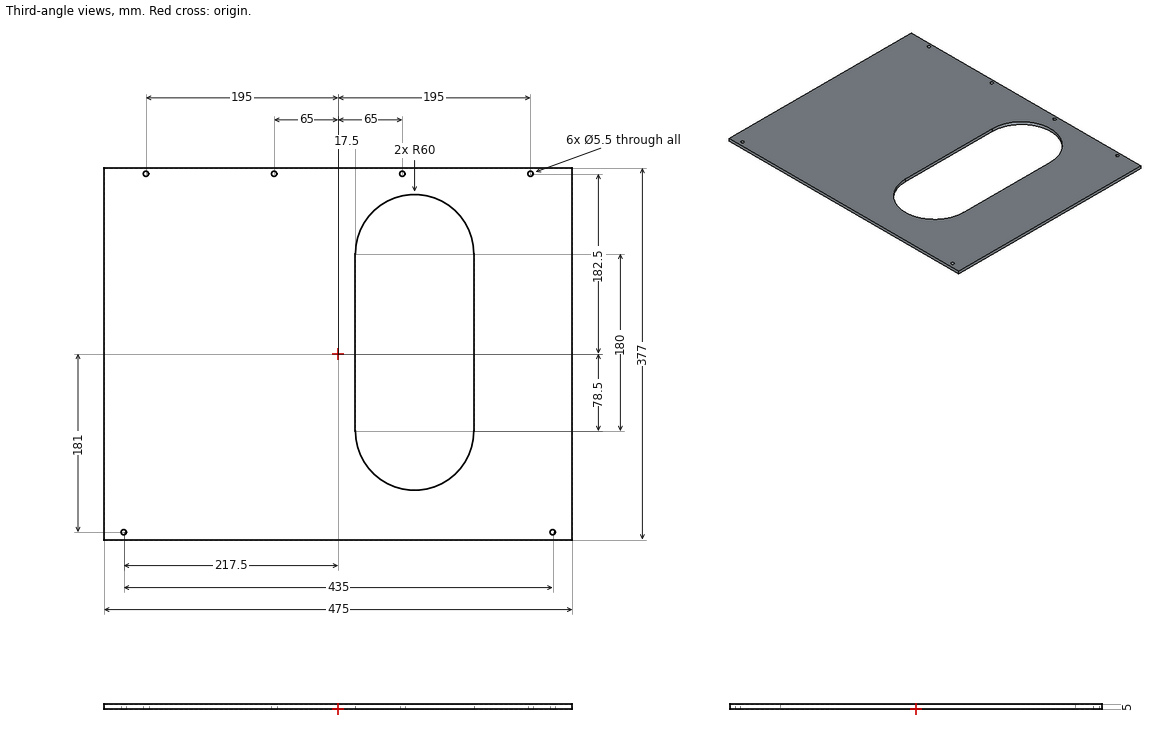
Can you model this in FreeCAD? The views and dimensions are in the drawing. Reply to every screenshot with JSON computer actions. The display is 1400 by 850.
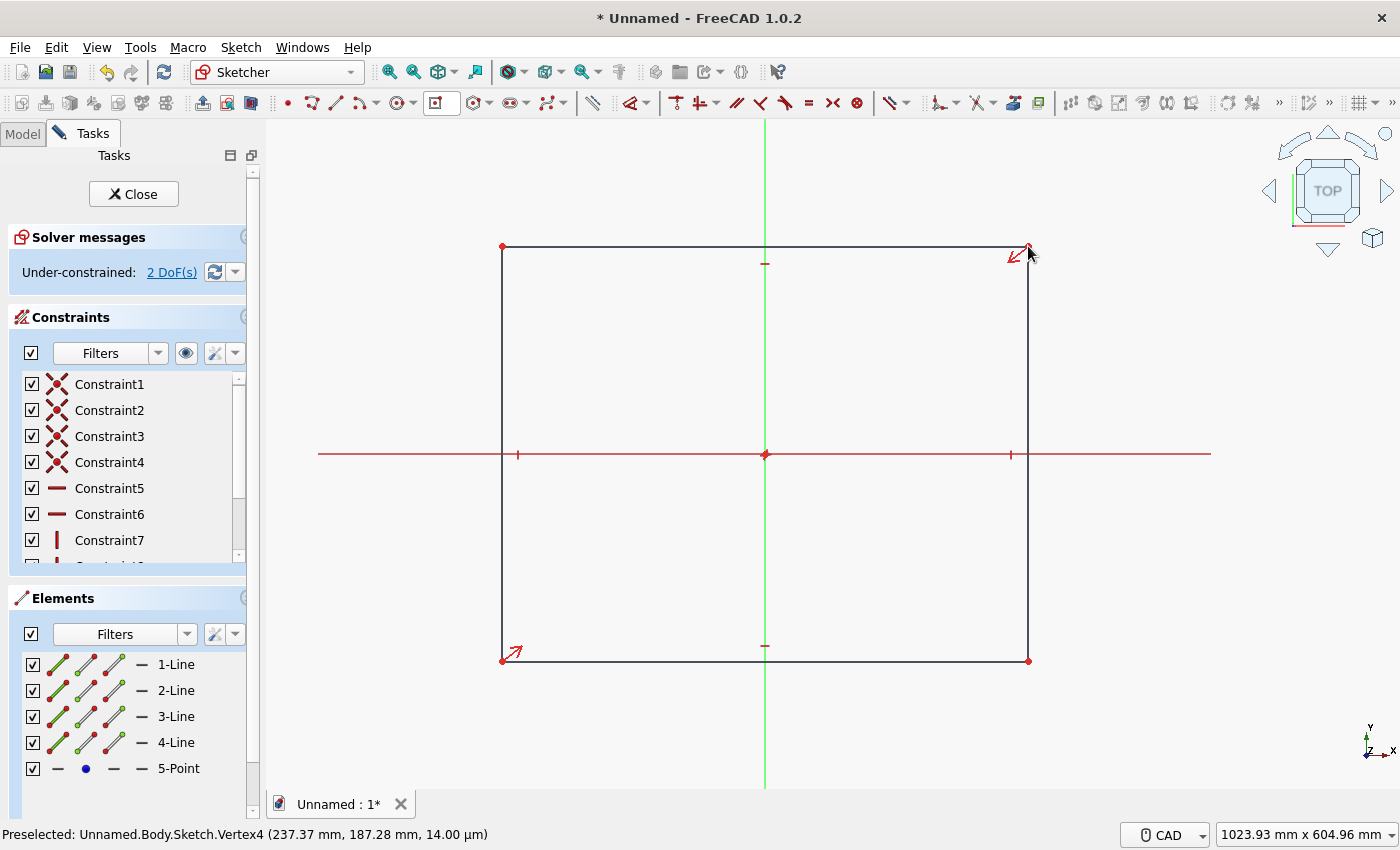
{"action": "left_click", "coordinate": [660, 662]}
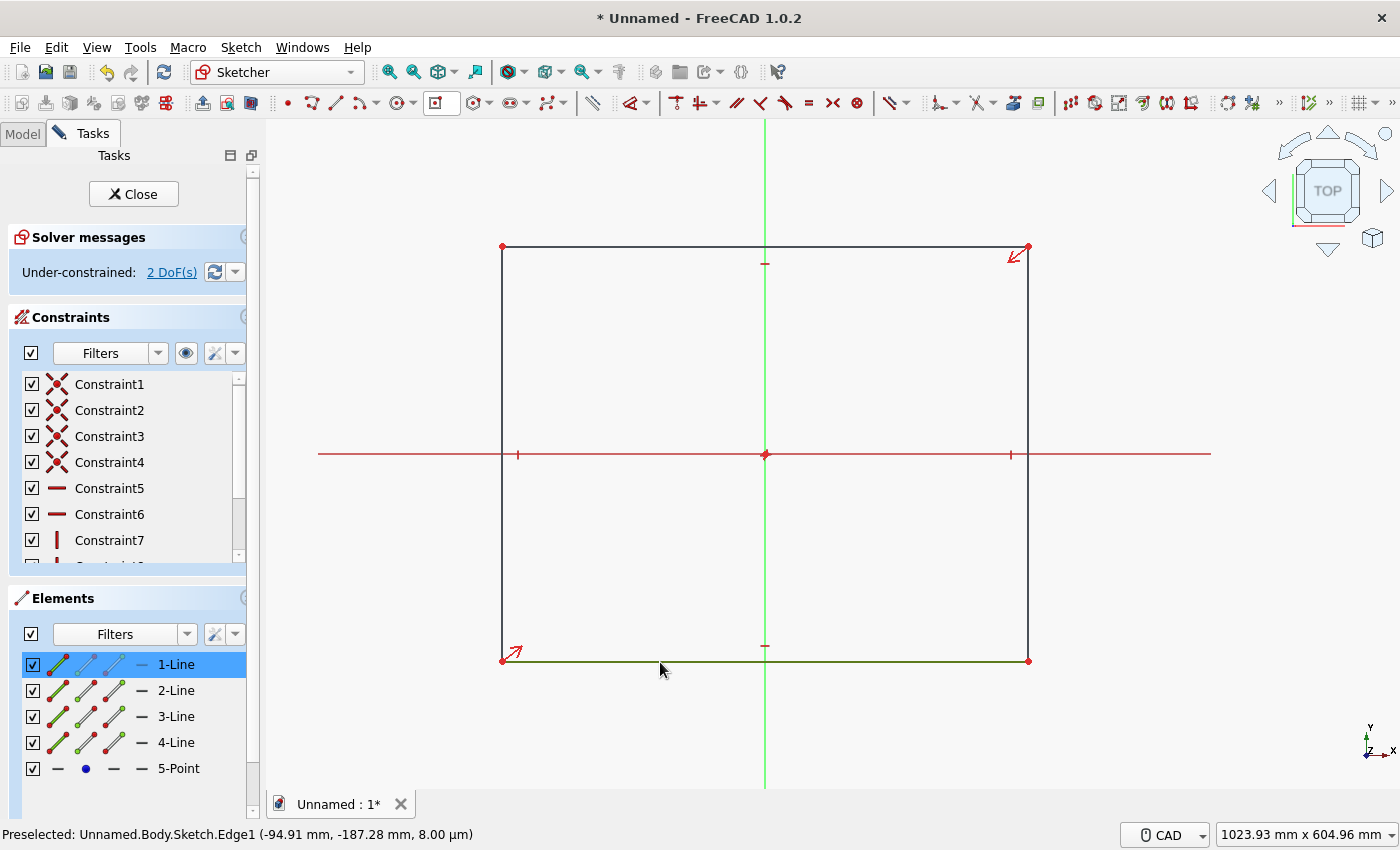
{"action": "key", "text": "l"}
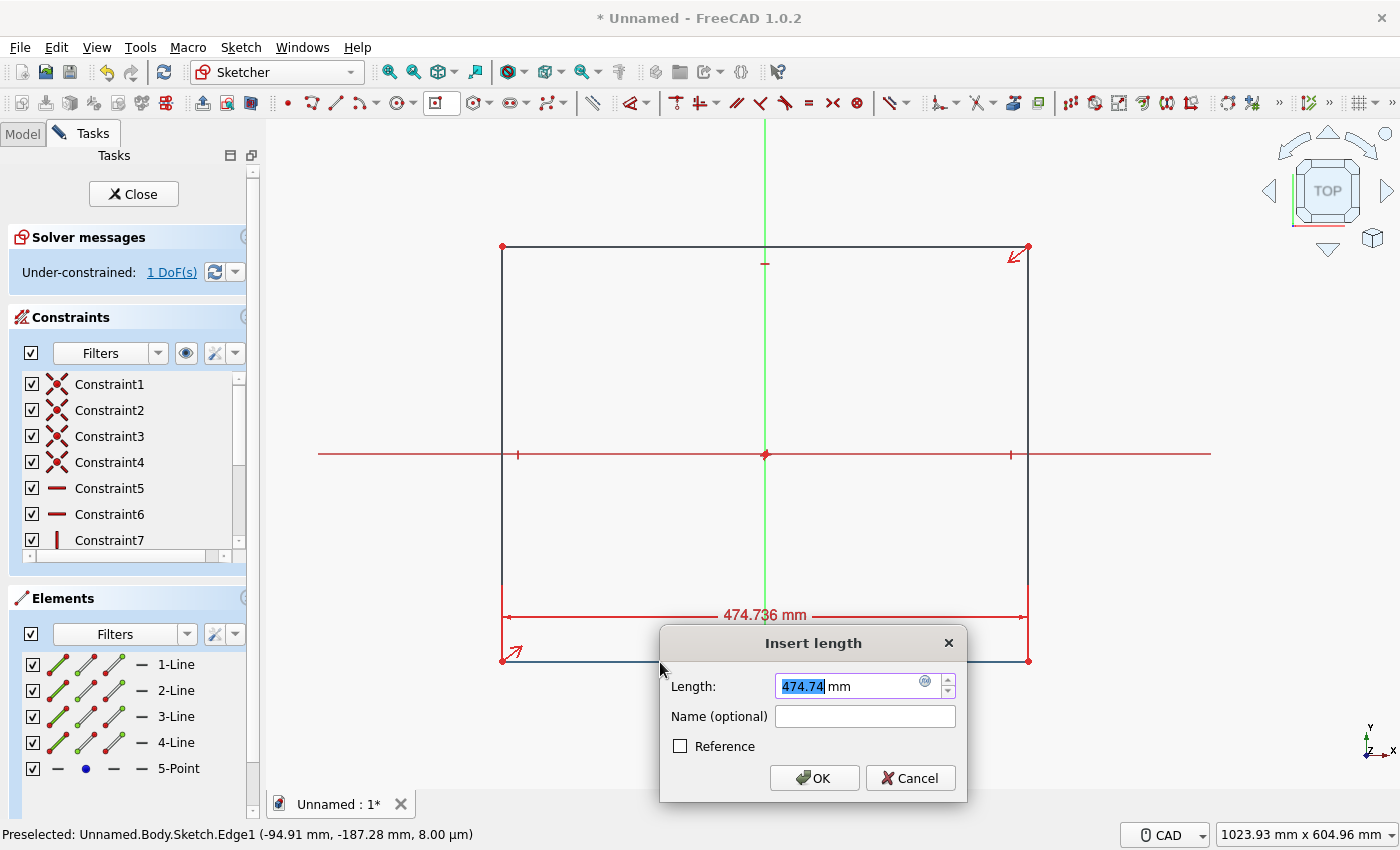
{"action": "type", "text": "475"}
{"action": "key", "text": "Return"}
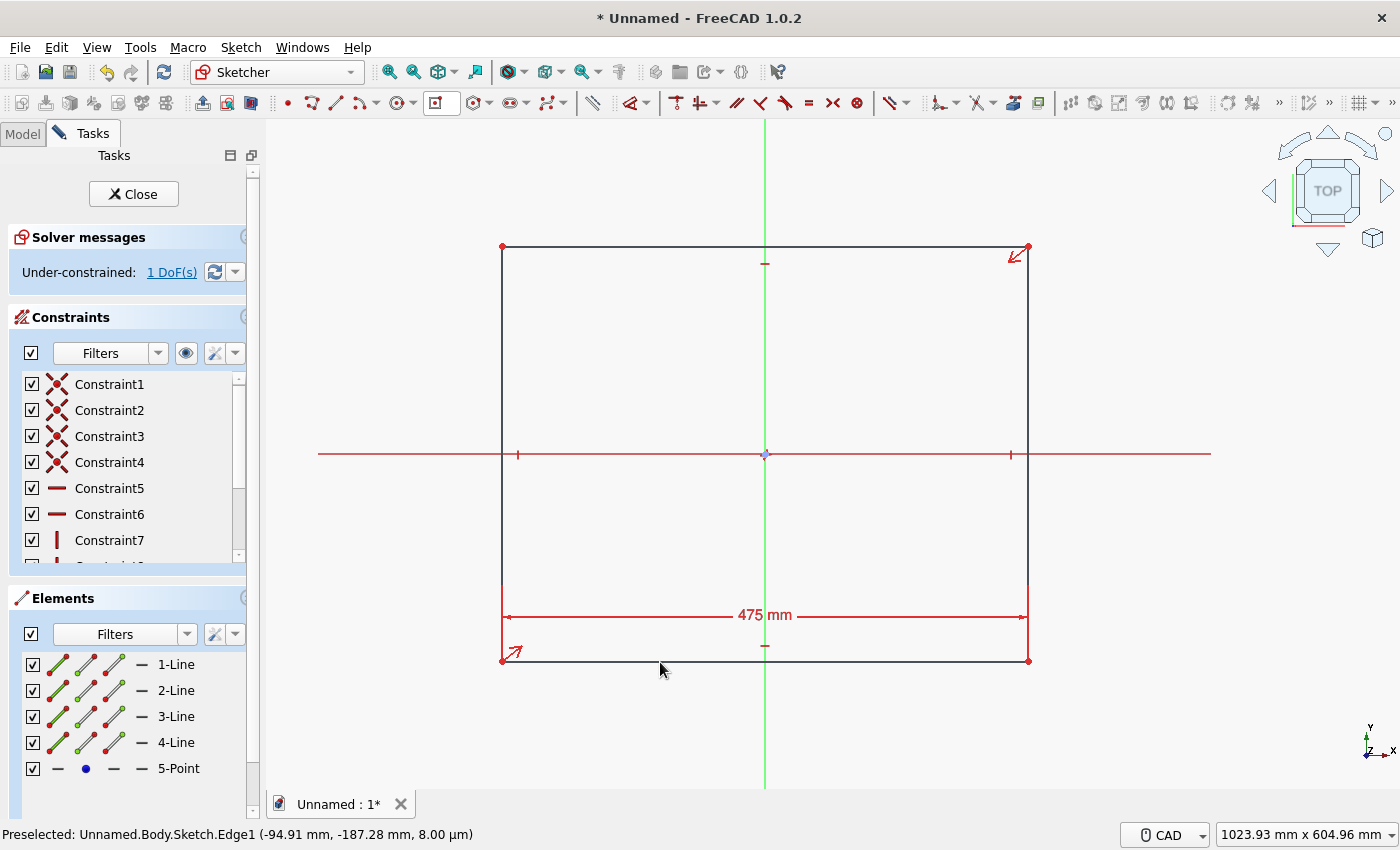
{"action": "left_click", "coordinate": [1028, 537]}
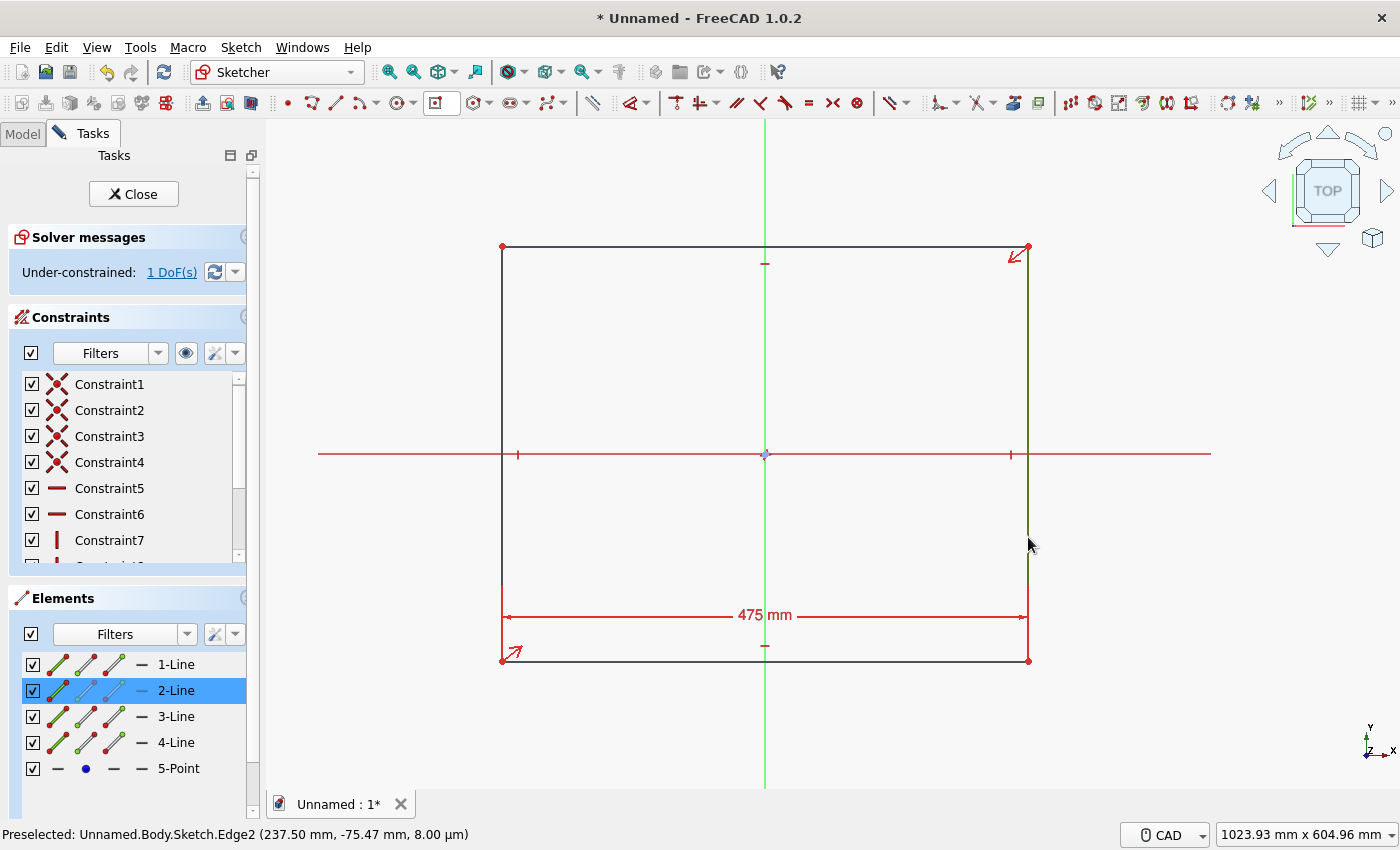
{"action": "key", "text": "i"}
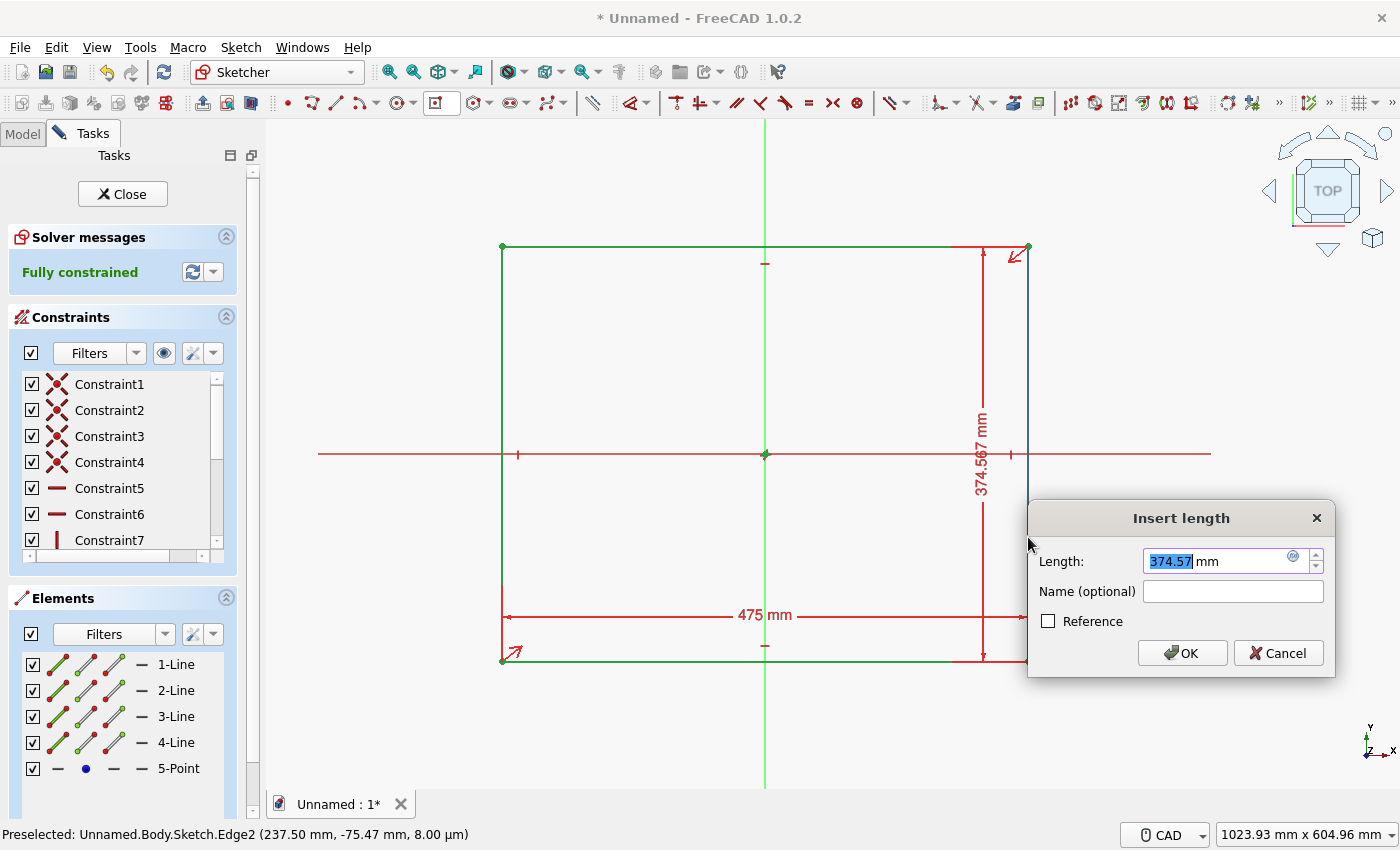
{"action": "type", "text": "377"}
{"action": "key", "text": "Return"}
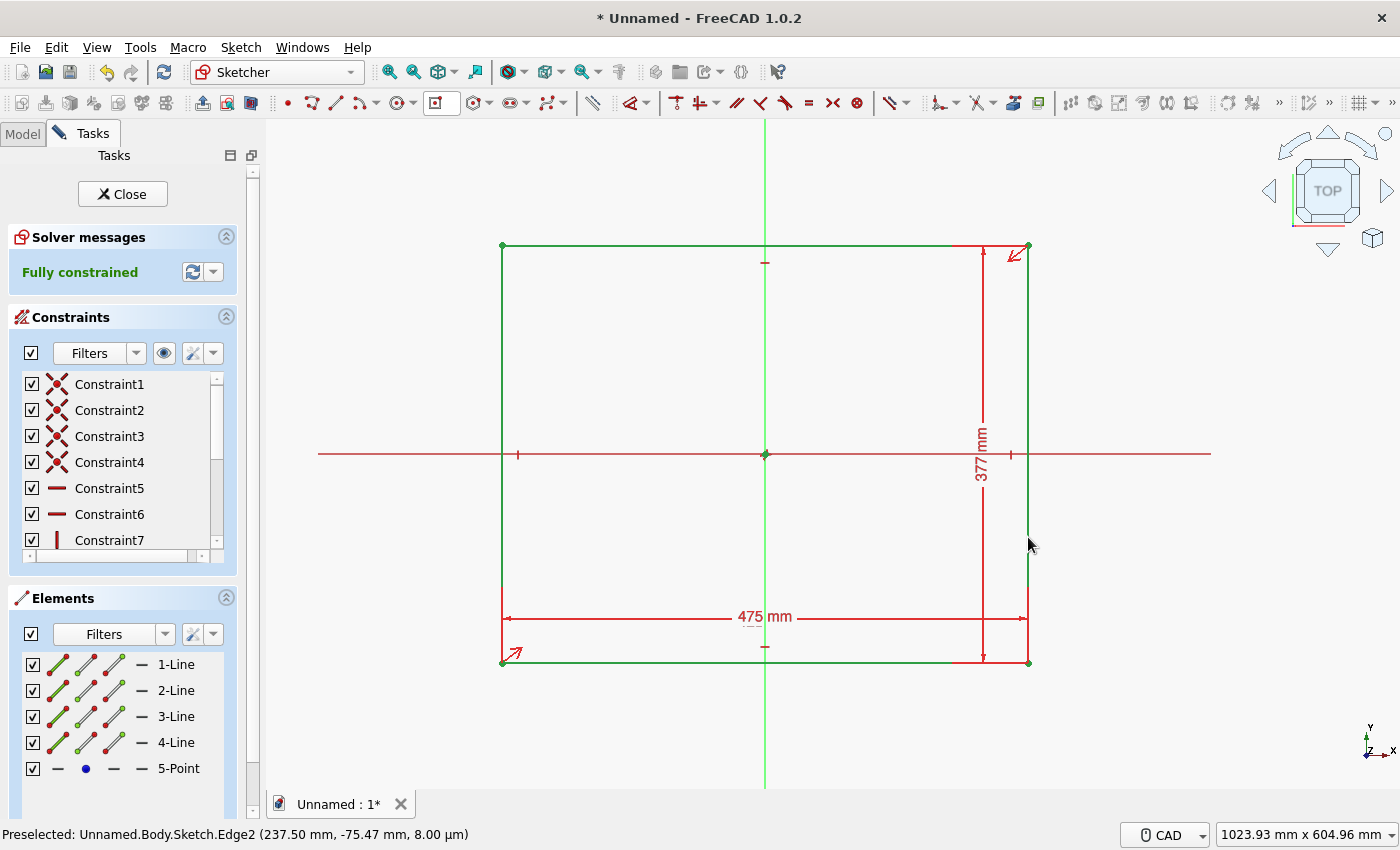
{"action": "left_click", "coordinate": [123, 194]}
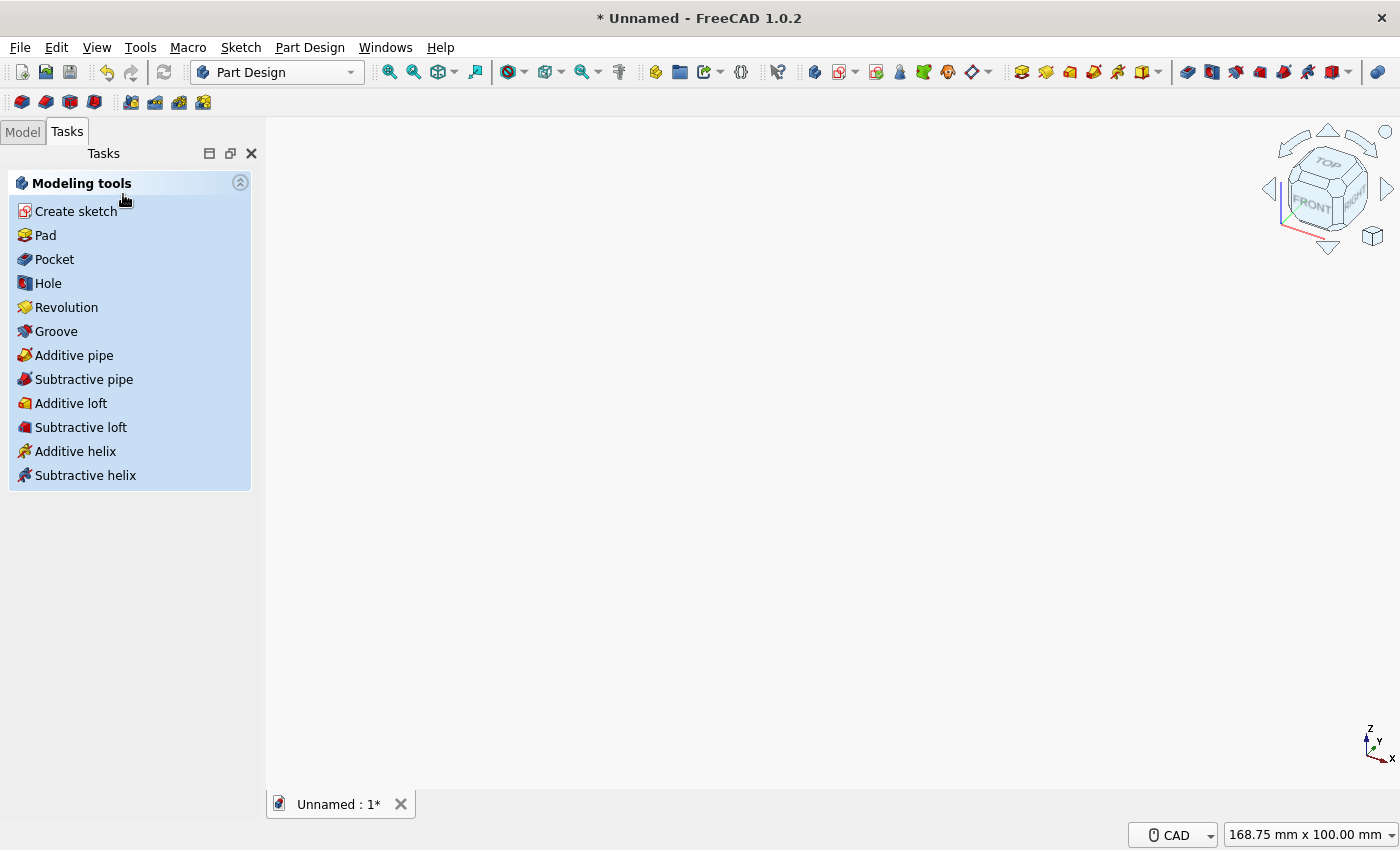
{"action": "left_click", "coordinate": [1022, 72]}